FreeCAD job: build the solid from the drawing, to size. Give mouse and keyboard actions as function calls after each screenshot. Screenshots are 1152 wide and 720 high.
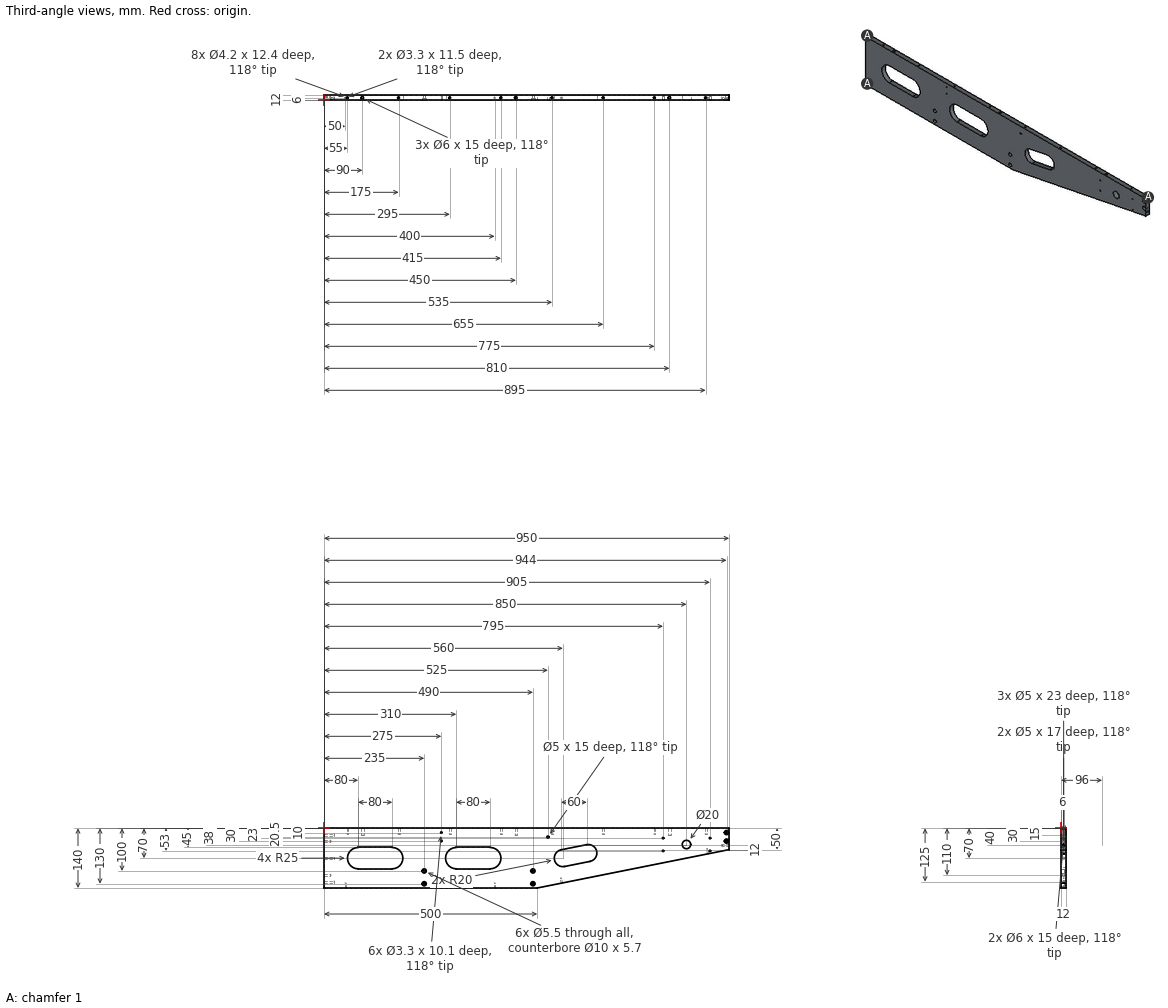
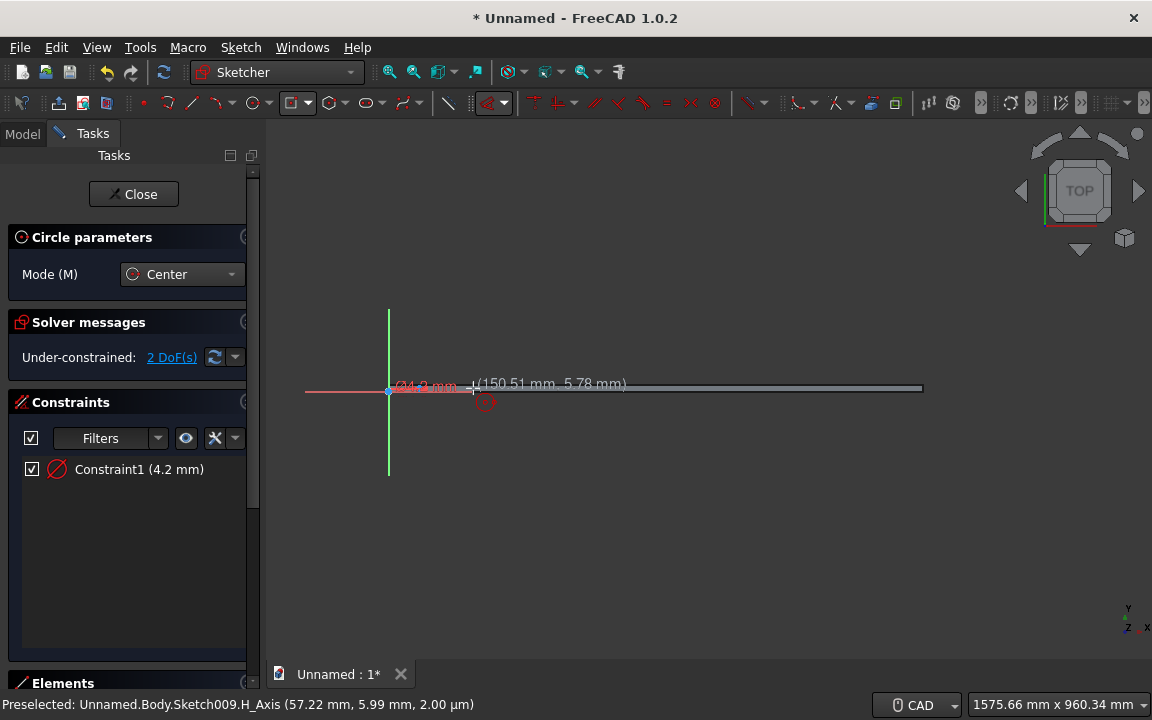
scroll(487, 388, up, 8)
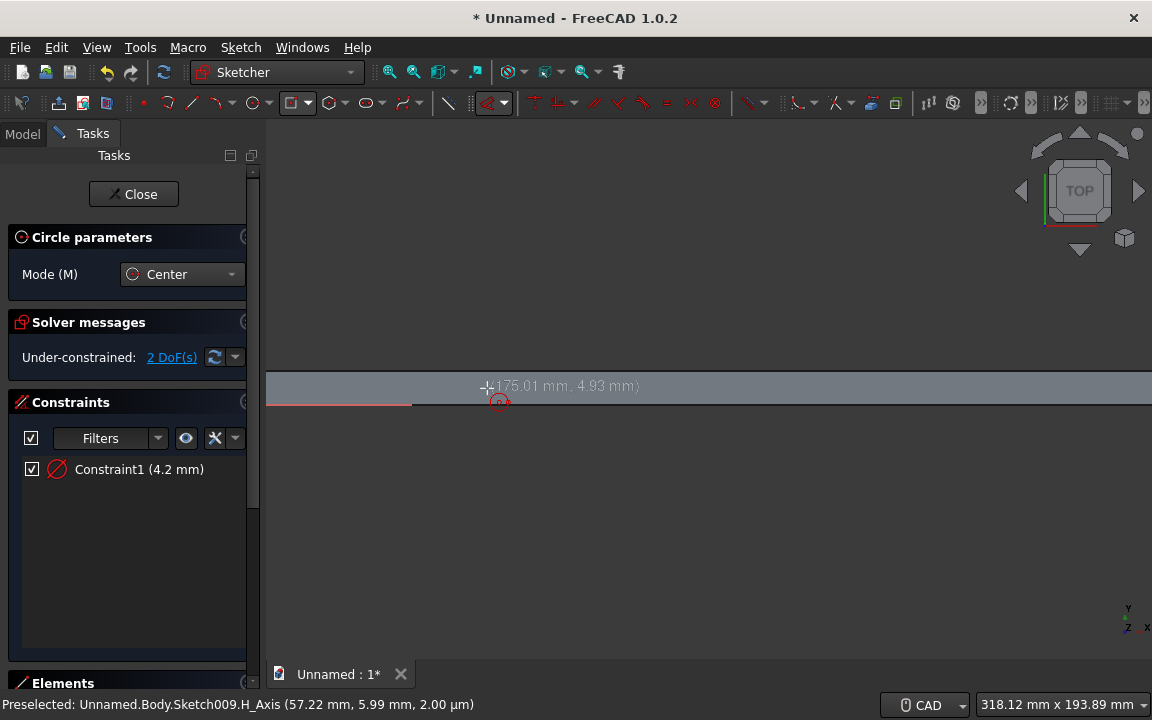
click(486, 388)
move(490, 384)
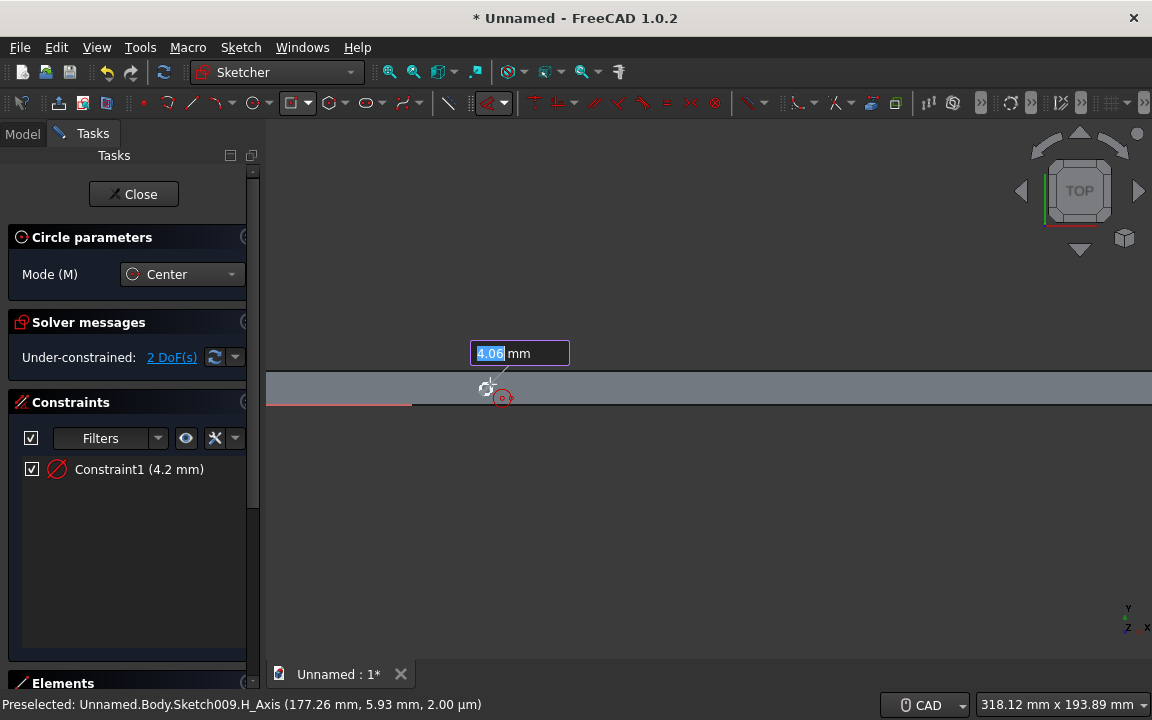
text(4.2)
key(Return)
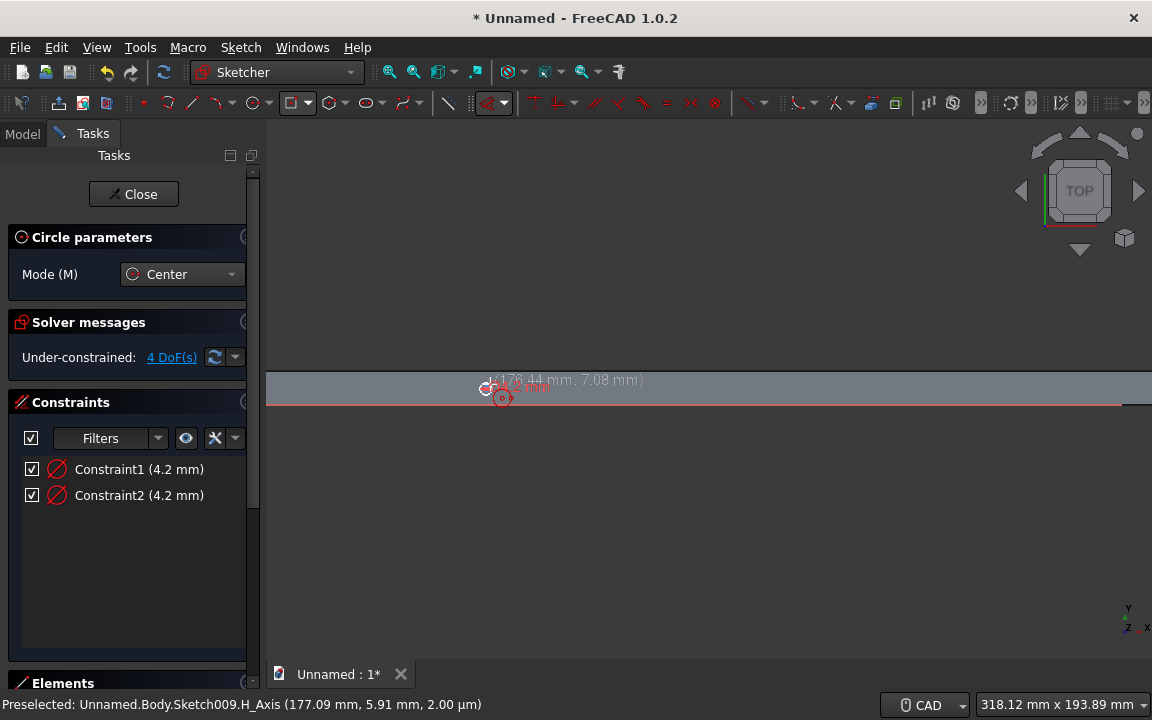
scroll(820, 388, up, 7)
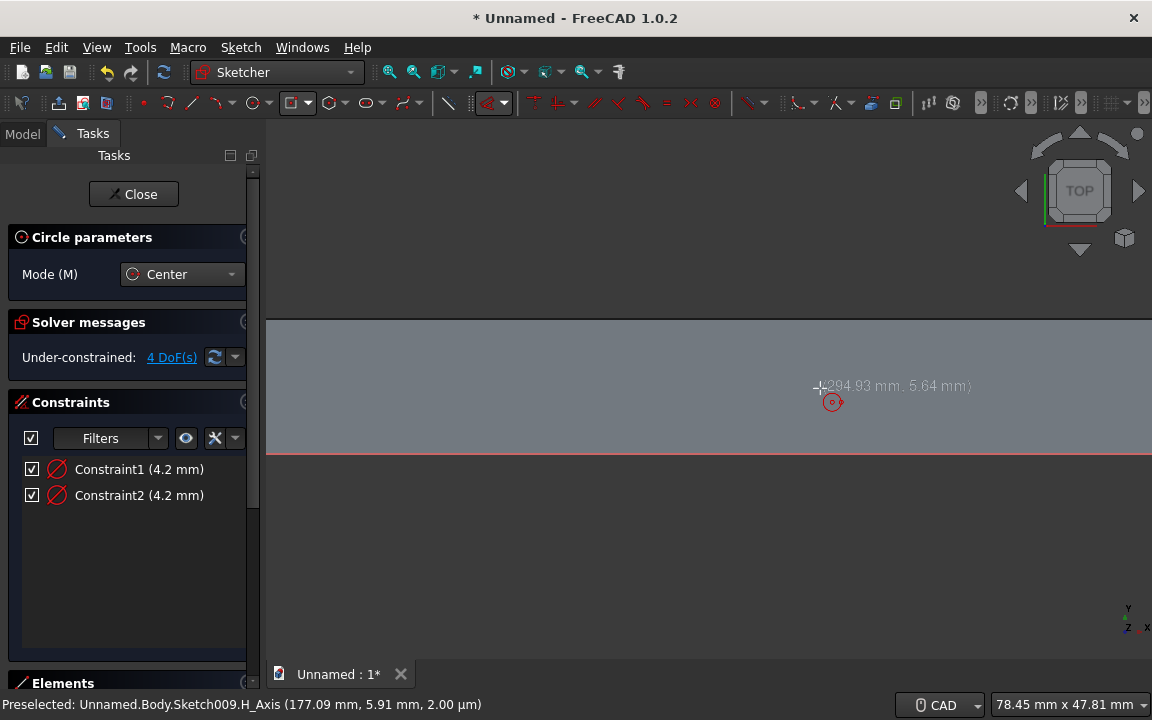
scroll(540, 388, down, 15)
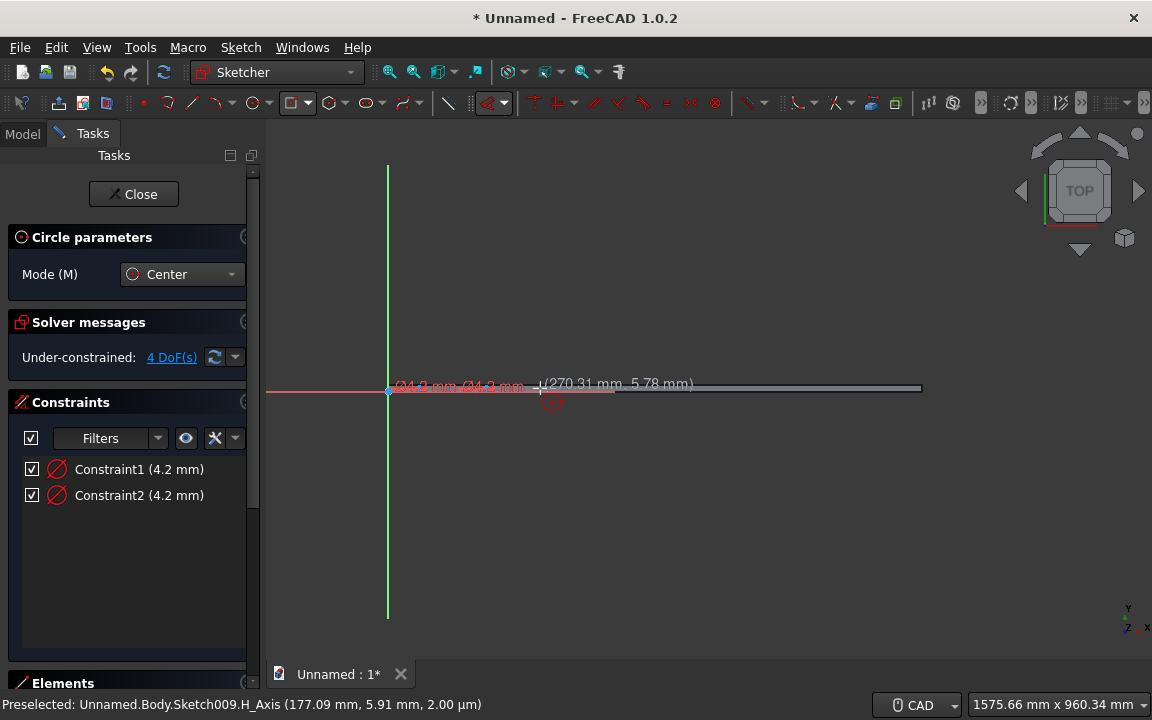
scroll(554, 388, up, 8)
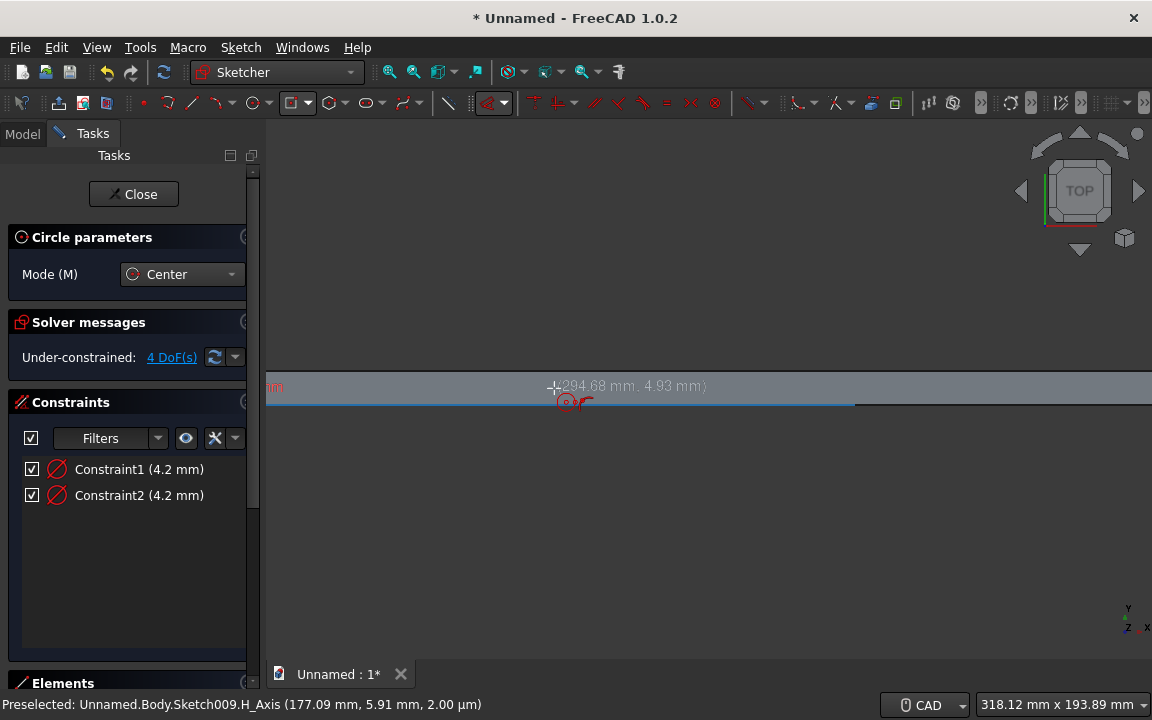
click(554, 388)
move(558, 384)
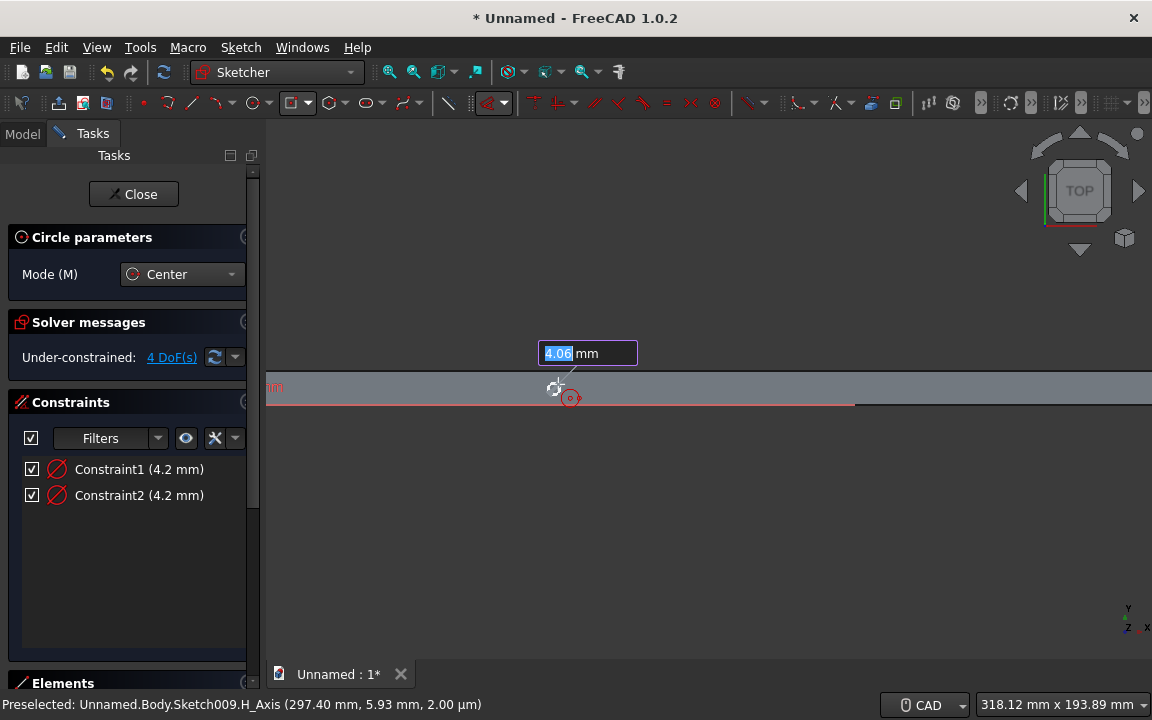
text(4.2)
key(Return)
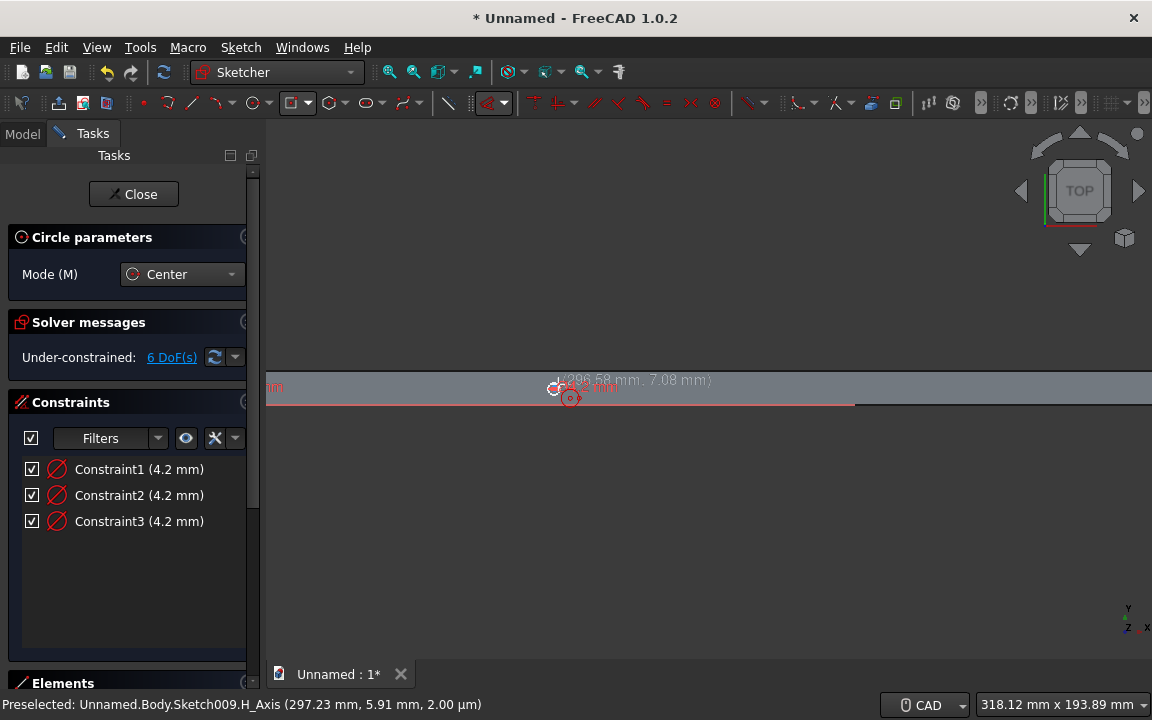
scroll(888, 388, up, 7)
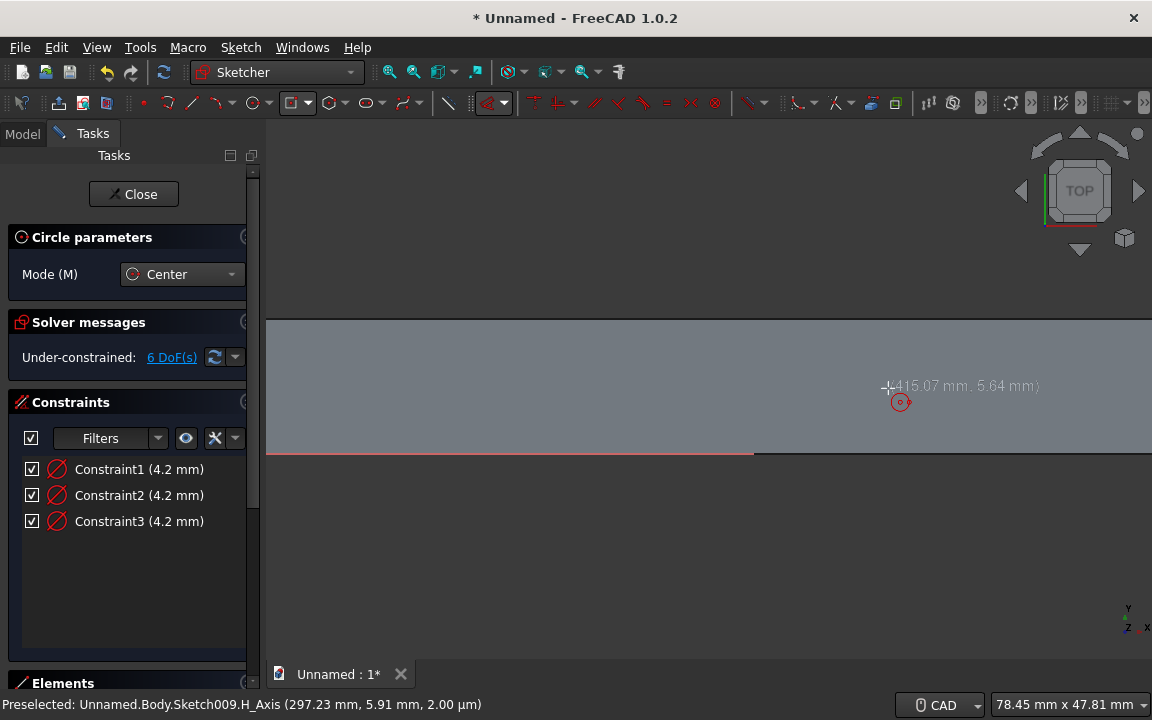
scroll(608, 388, down, 15)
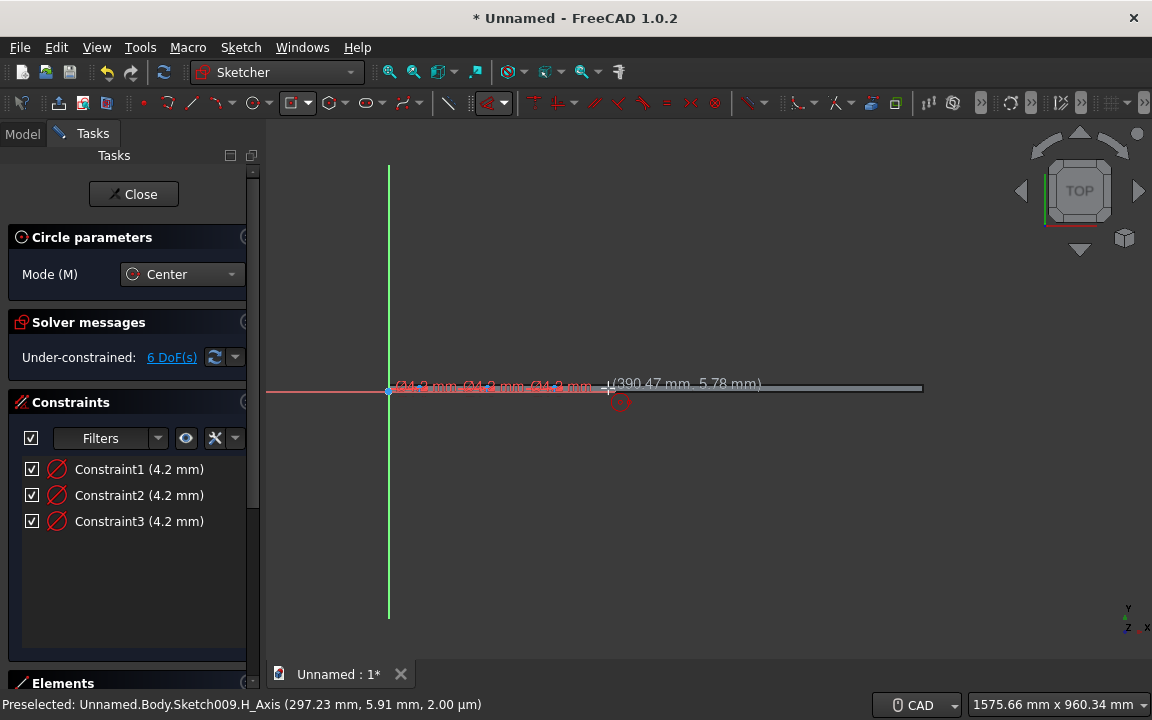
scroll(622, 388, up, 8)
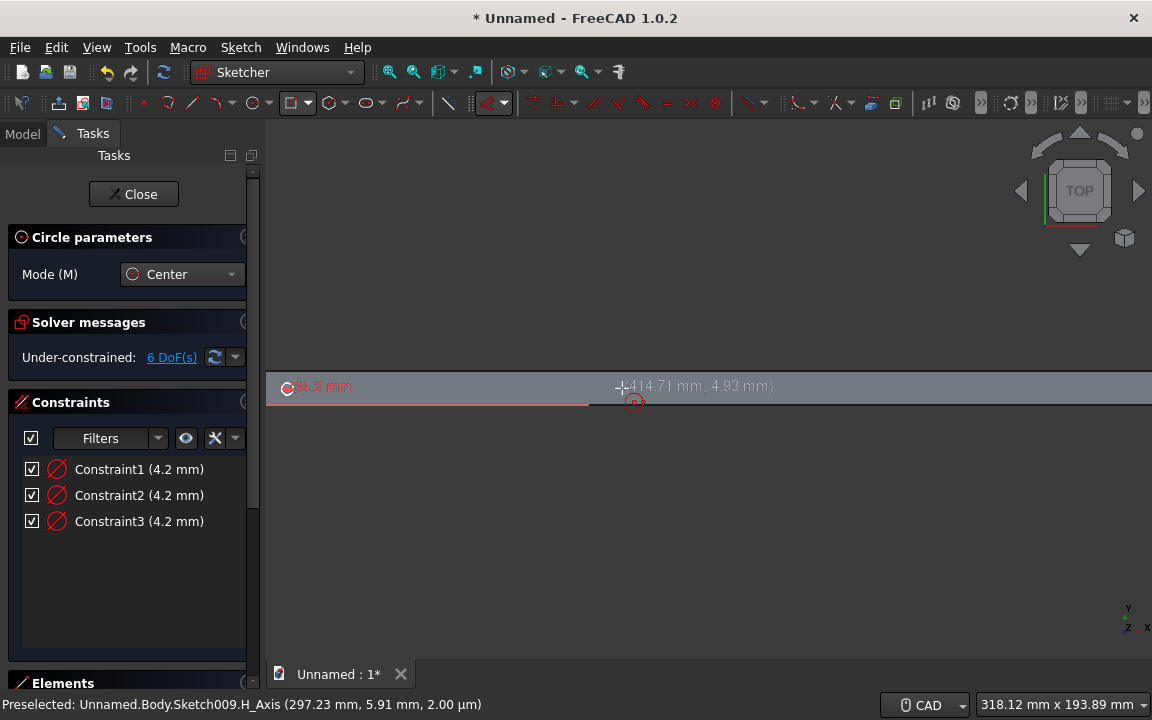
click(621, 388)
move(625, 384)